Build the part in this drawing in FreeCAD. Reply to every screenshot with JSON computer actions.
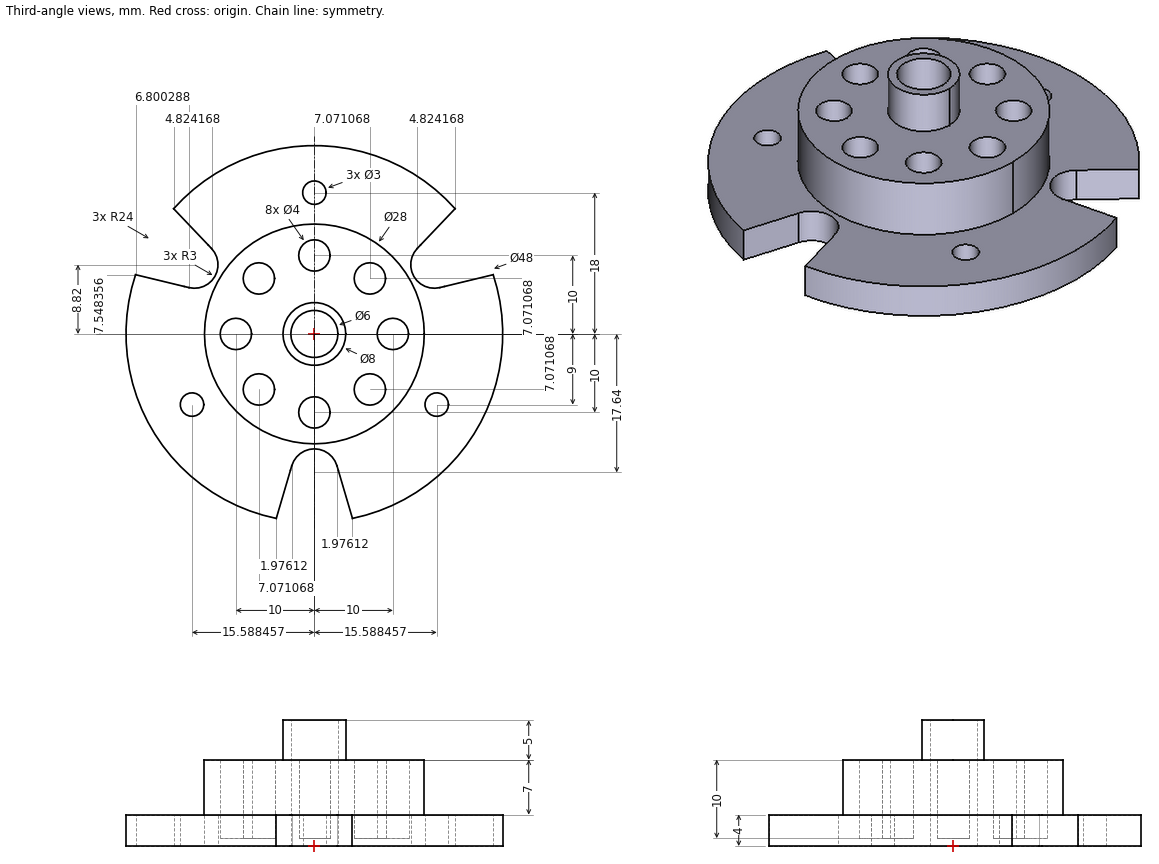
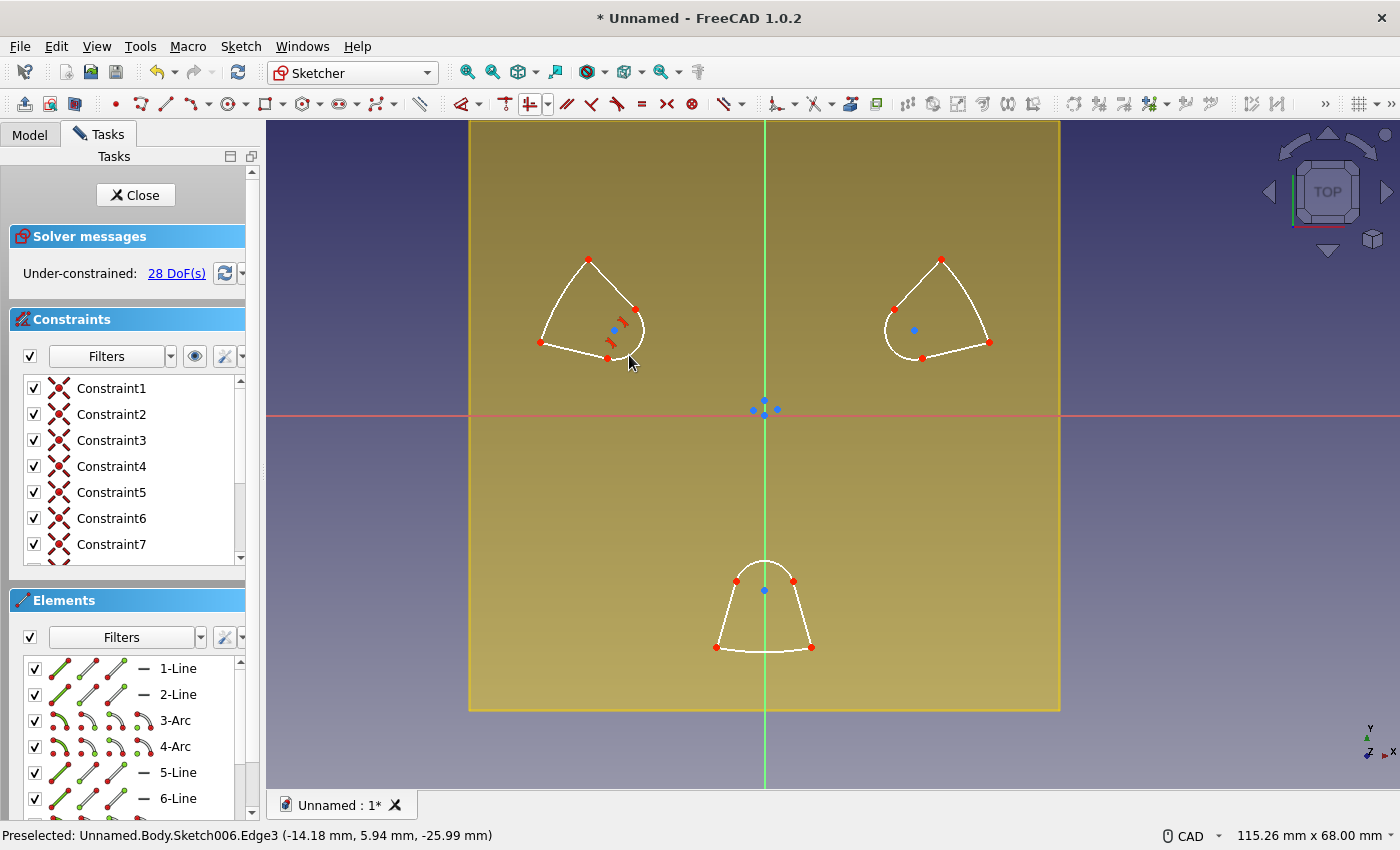
{"action": "left_click", "coordinate": [927, 275]}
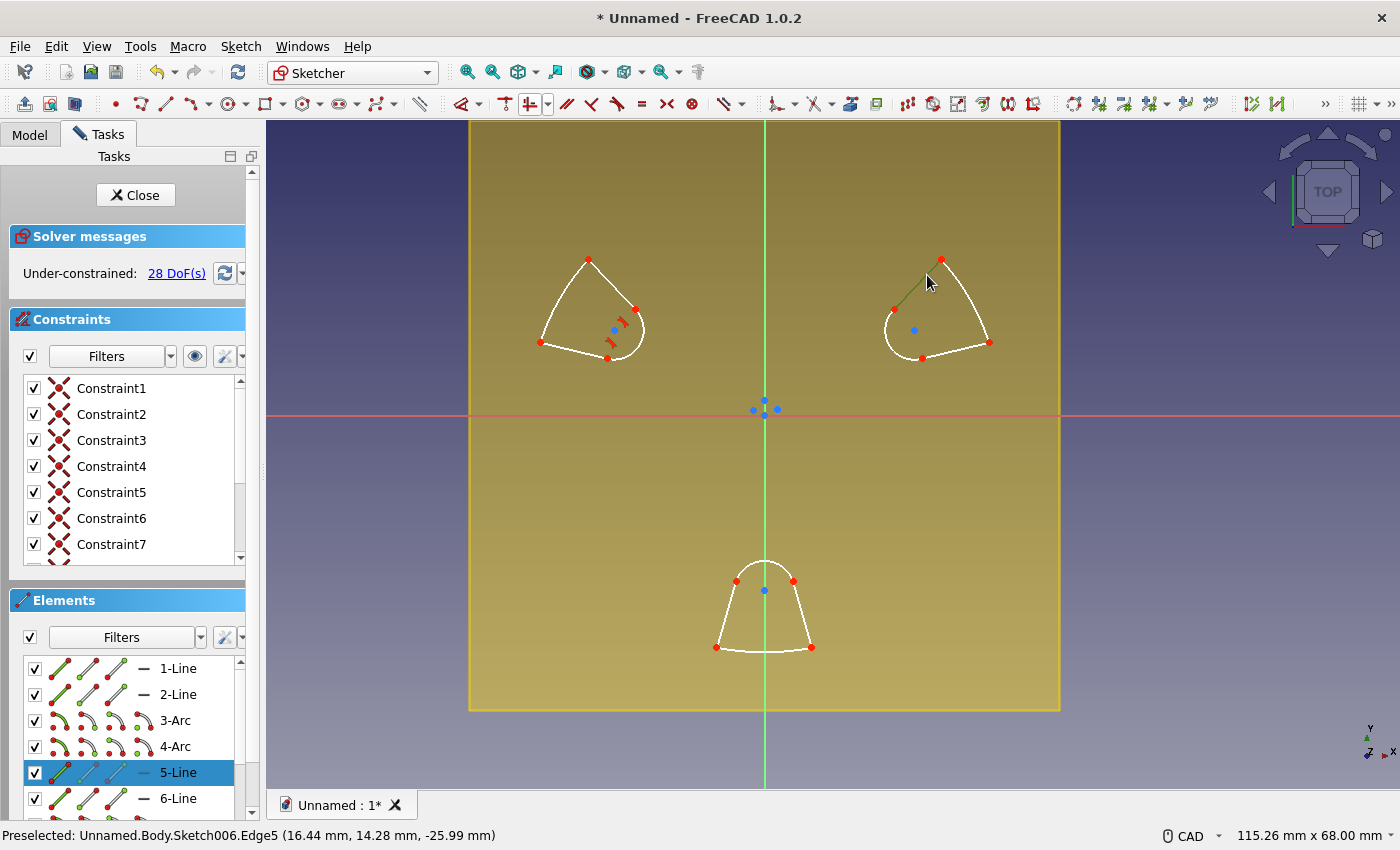
{"action": "left_click", "coordinate": [885, 330]}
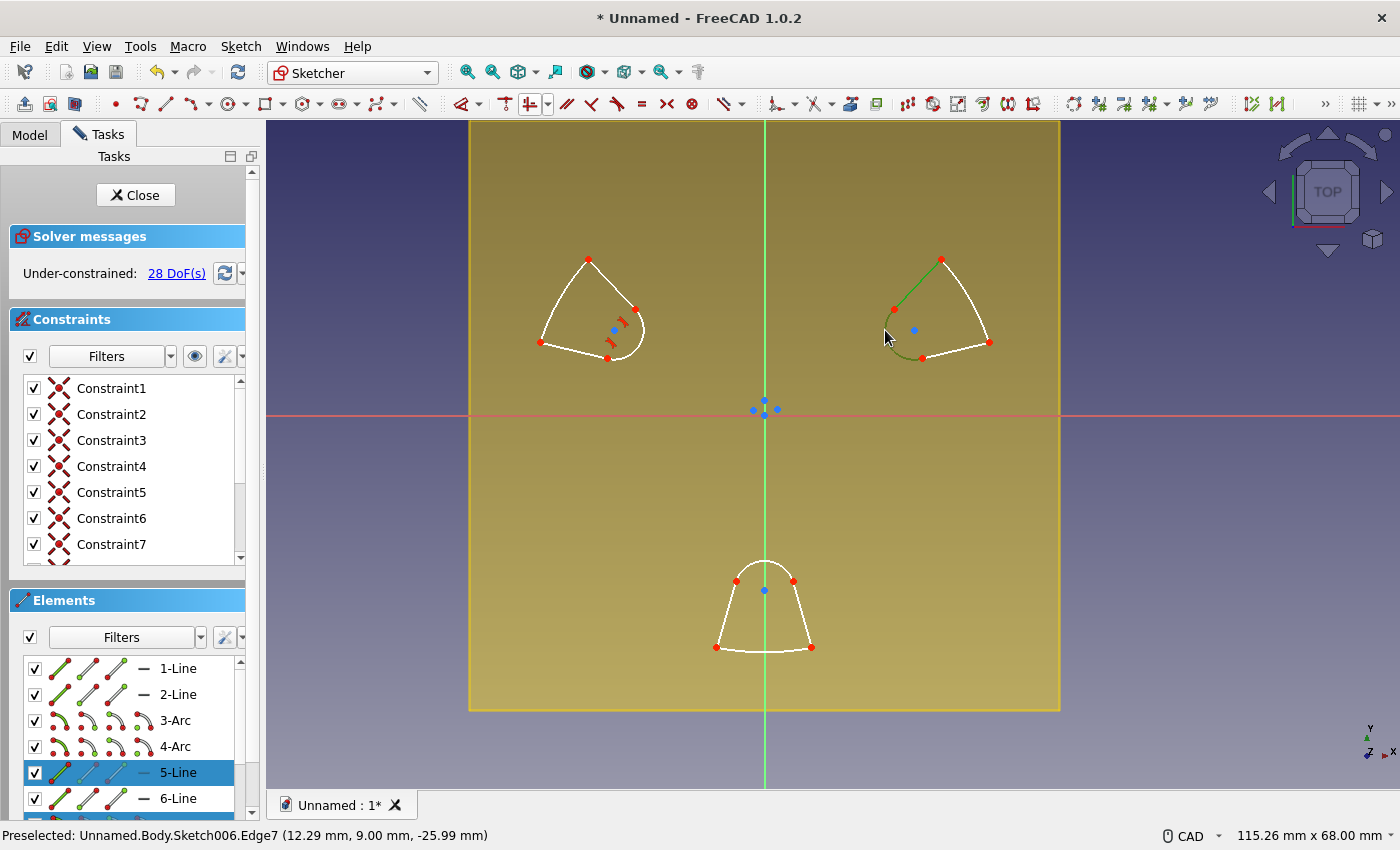
{"action": "left_click", "coordinate": [617, 104]}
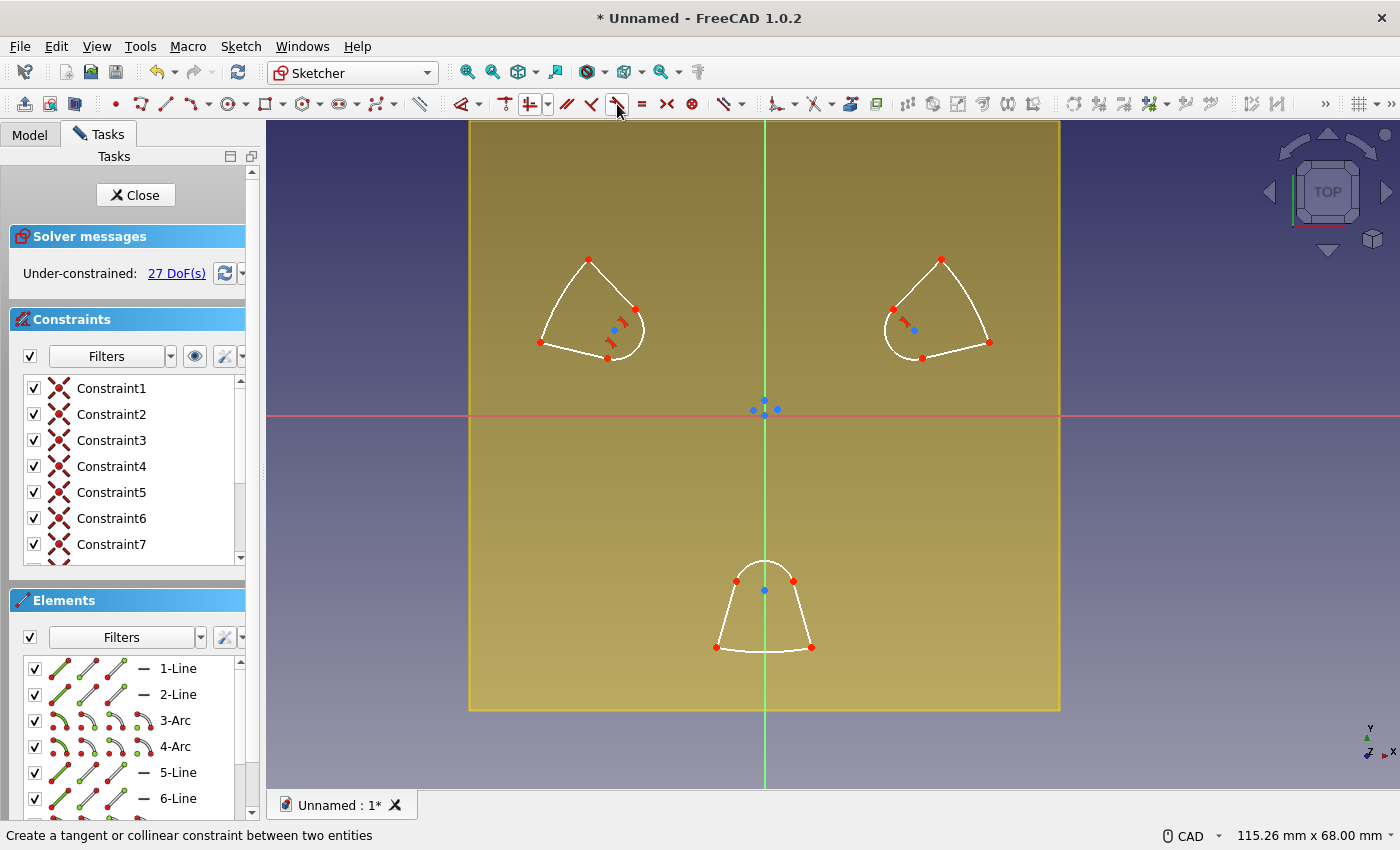
{"action": "left_click", "coordinate": [942, 354]}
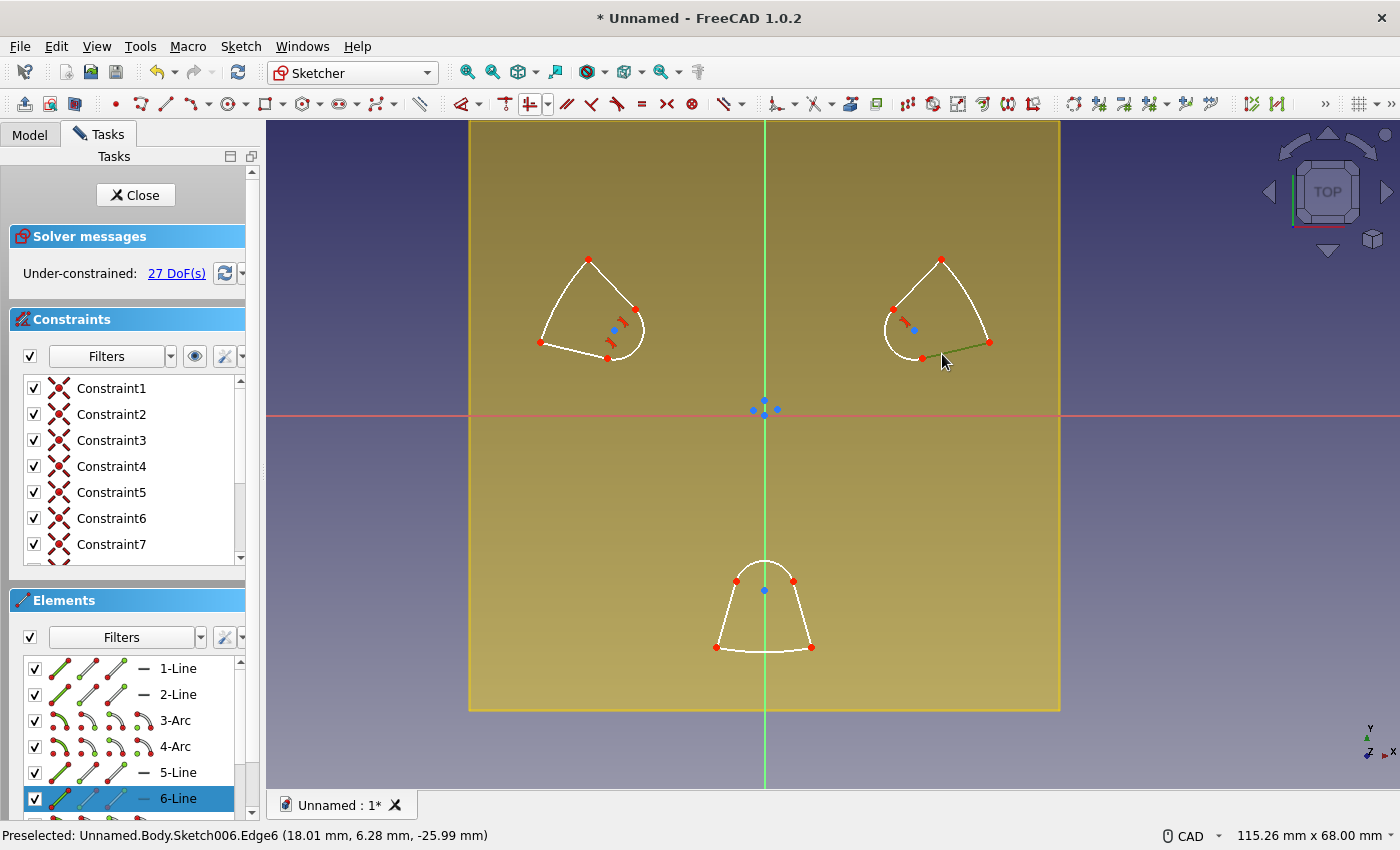
{"action": "left_click", "coordinate": [885, 331]}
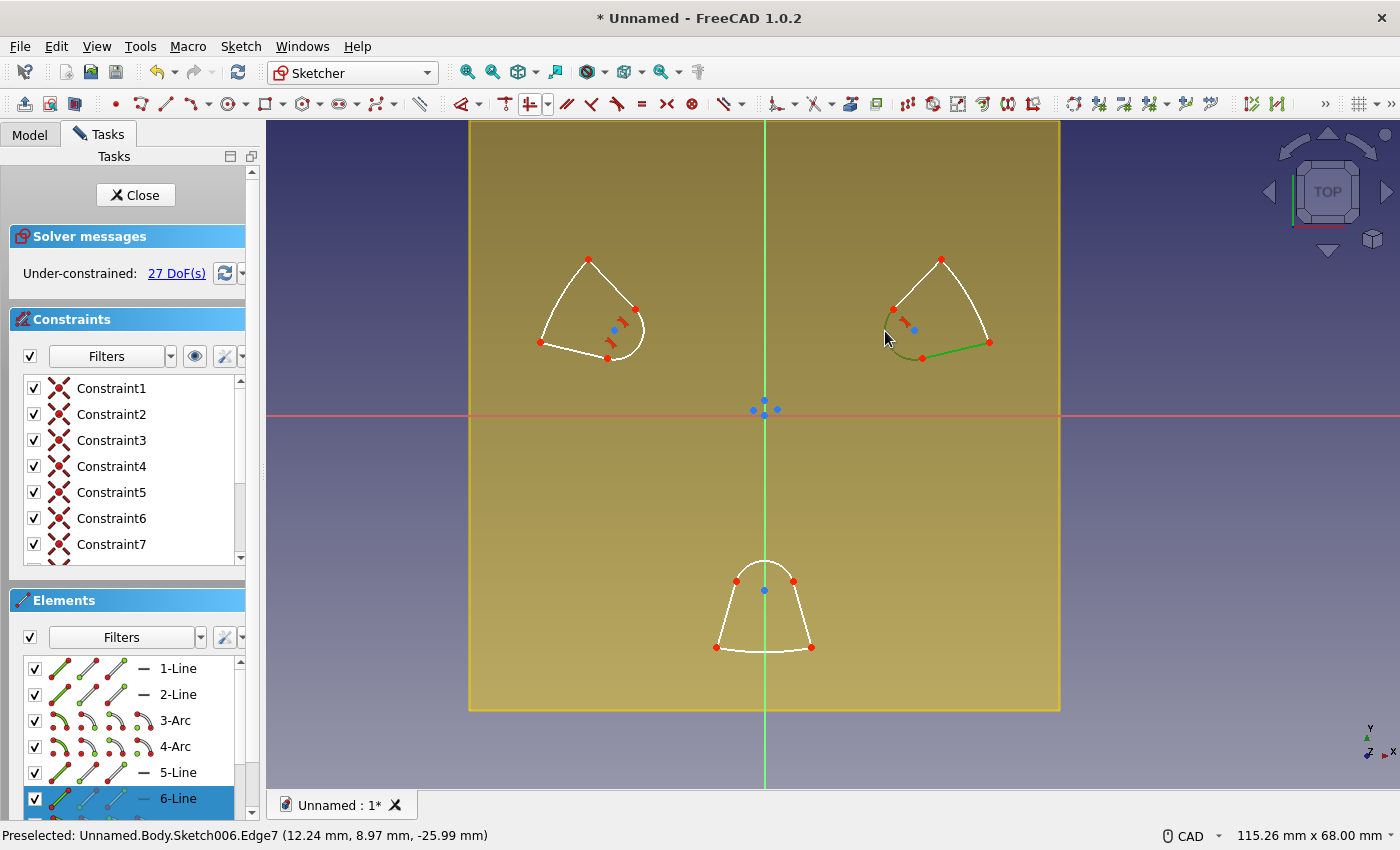
{"action": "key", "text": "t"}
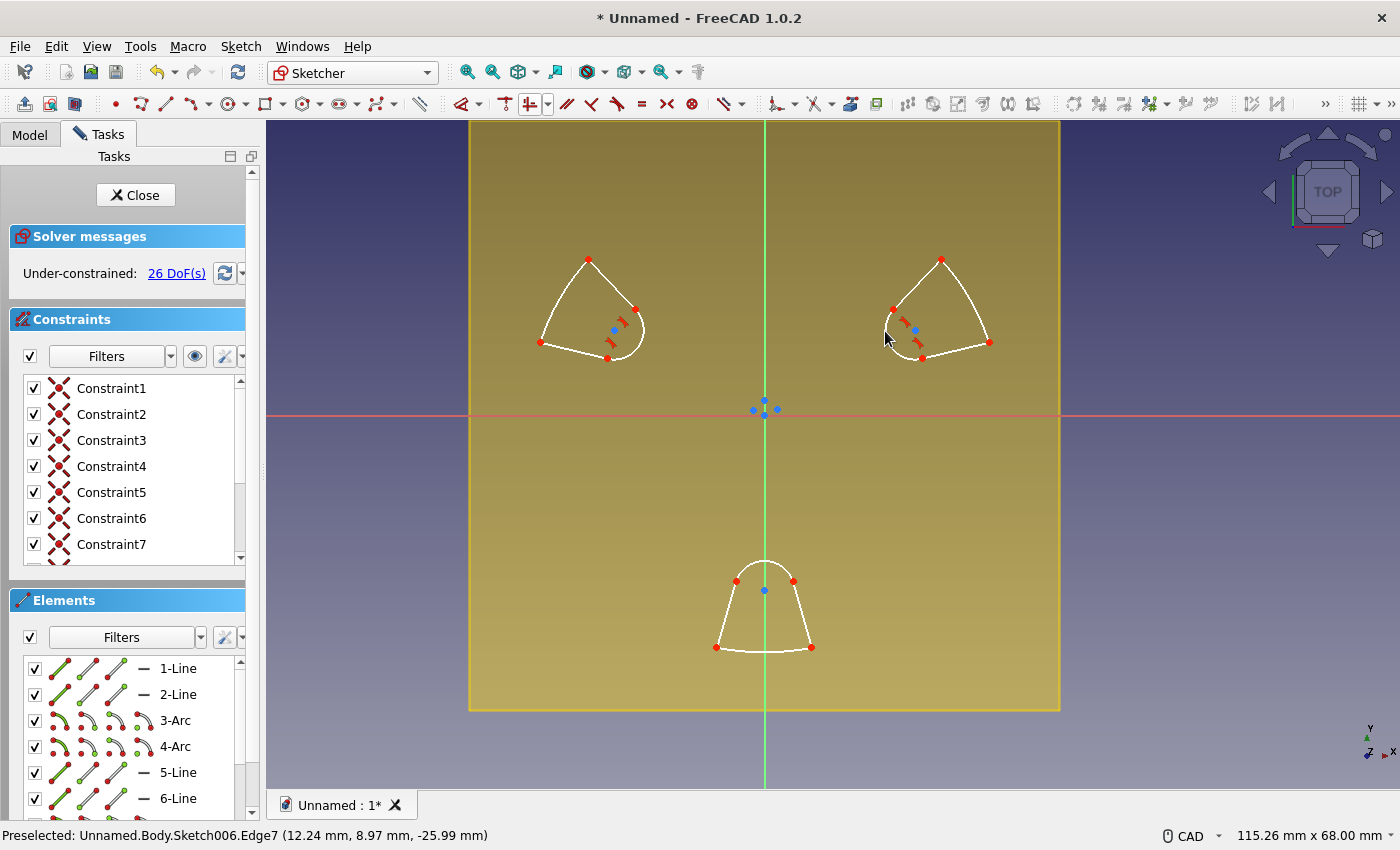
{"action": "left_click", "coordinate": [806, 628]}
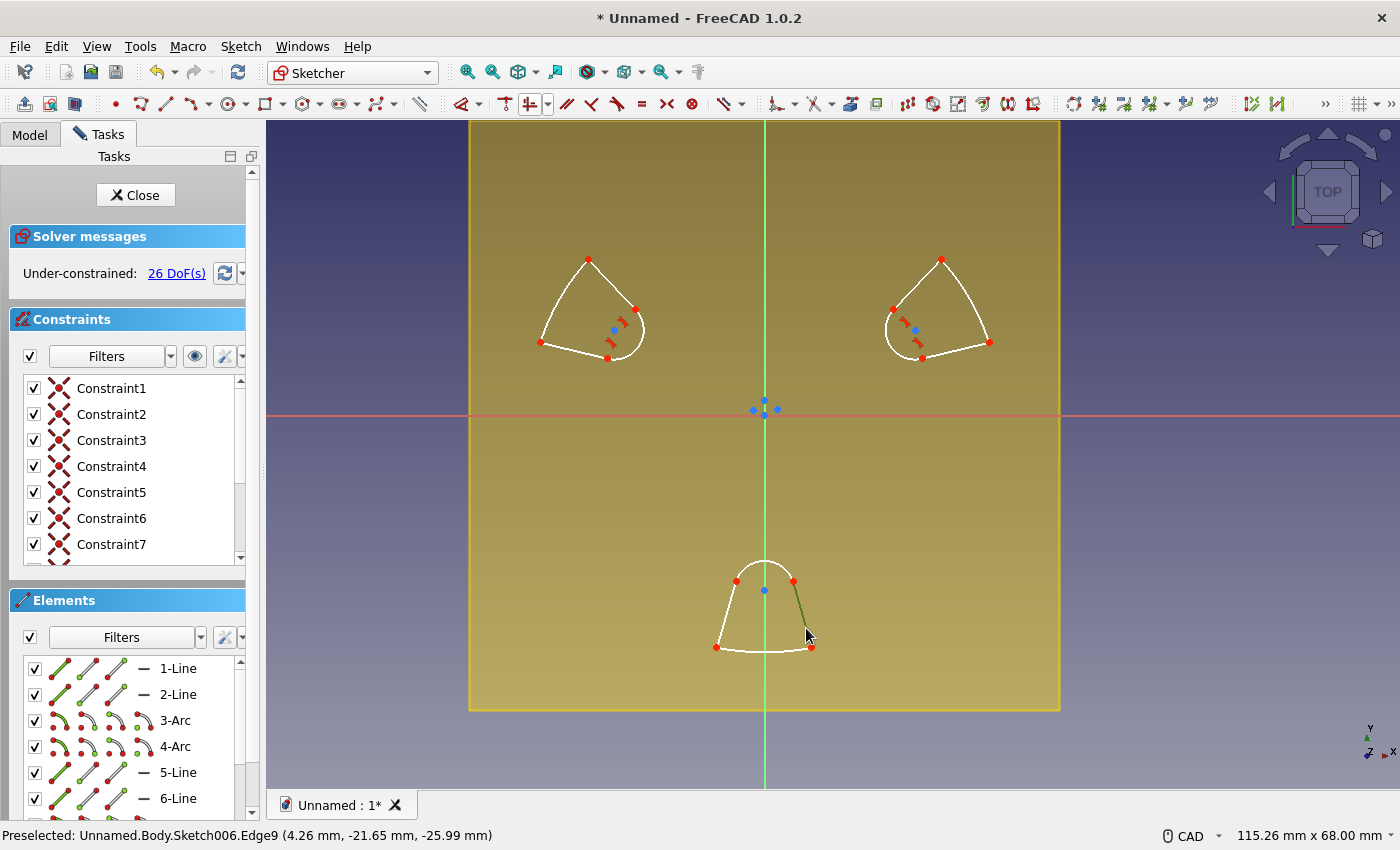
{"action": "left_click", "coordinate": [779, 565]}